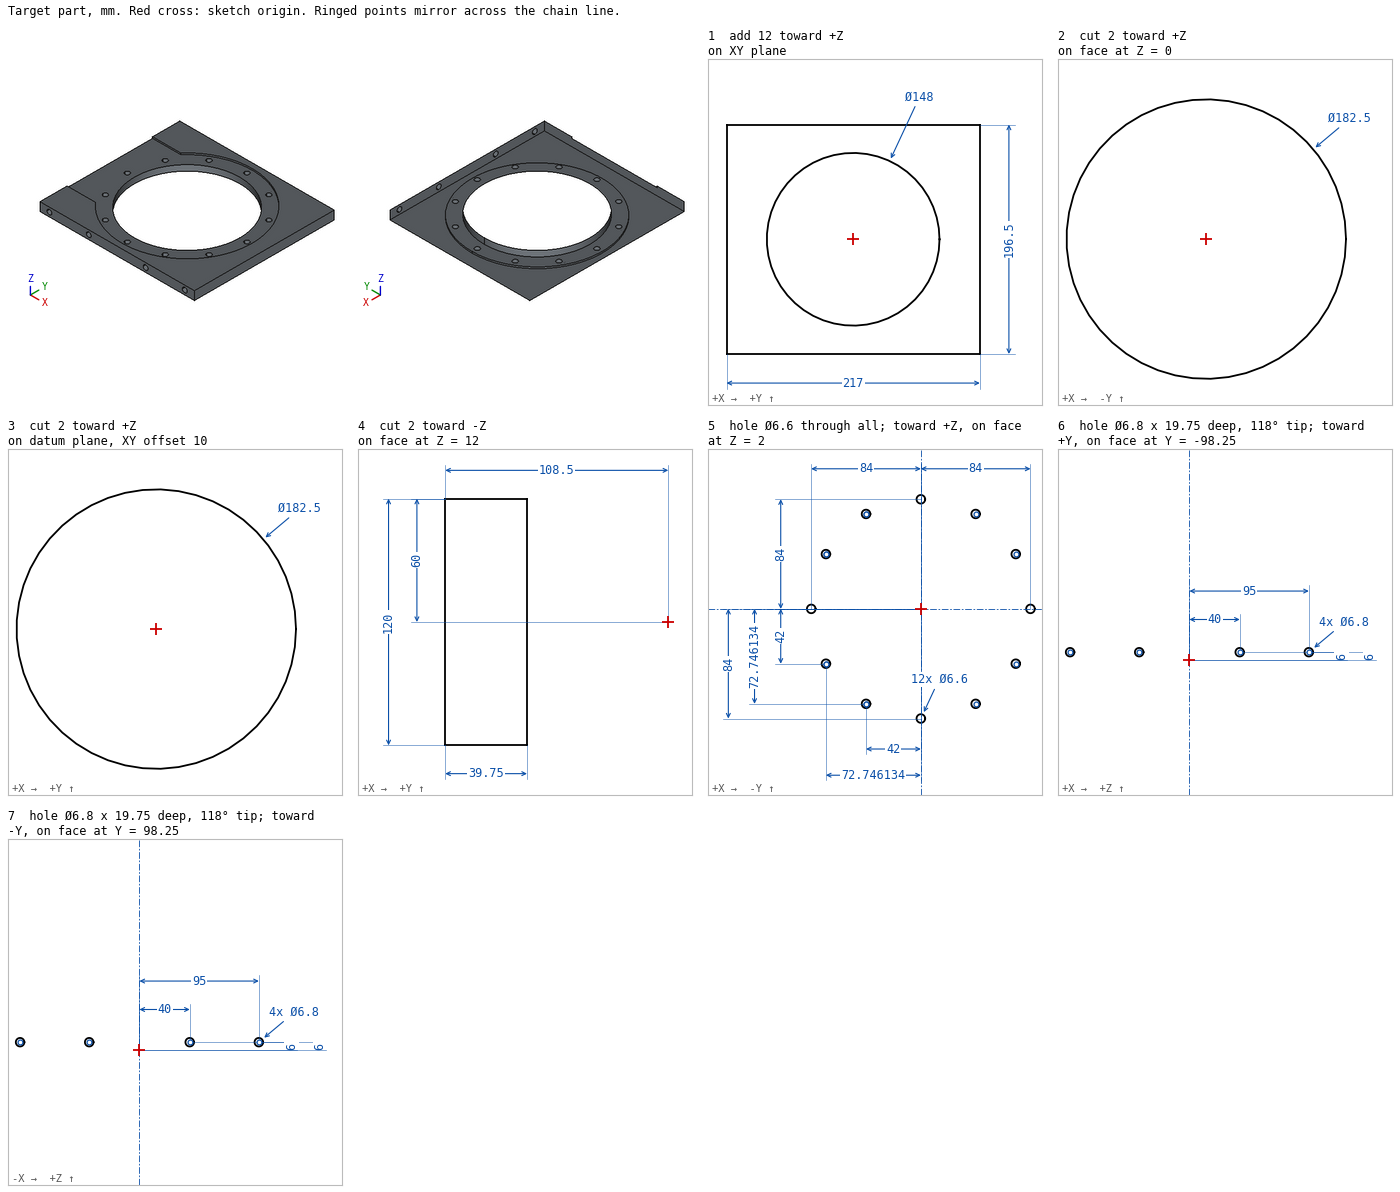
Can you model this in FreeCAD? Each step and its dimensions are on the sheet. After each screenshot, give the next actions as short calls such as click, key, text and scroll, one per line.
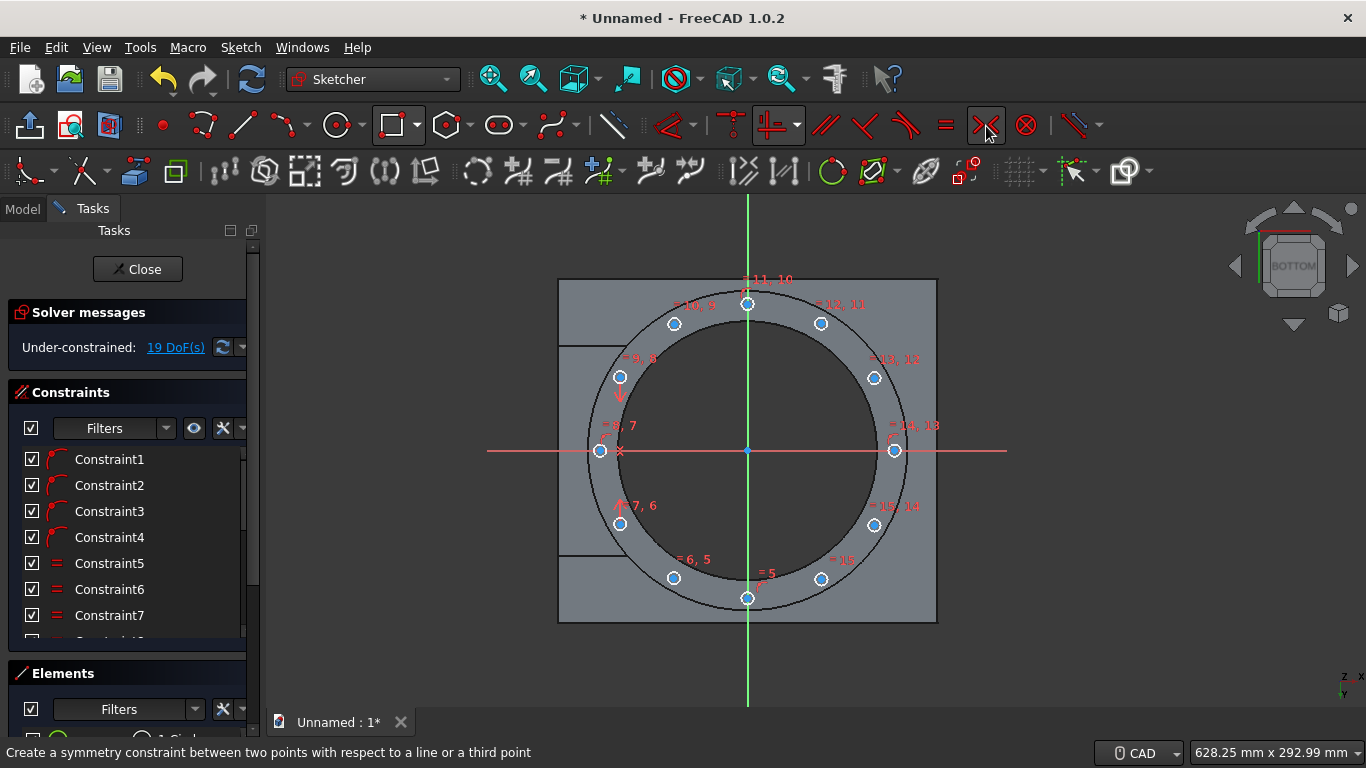
click(674, 578)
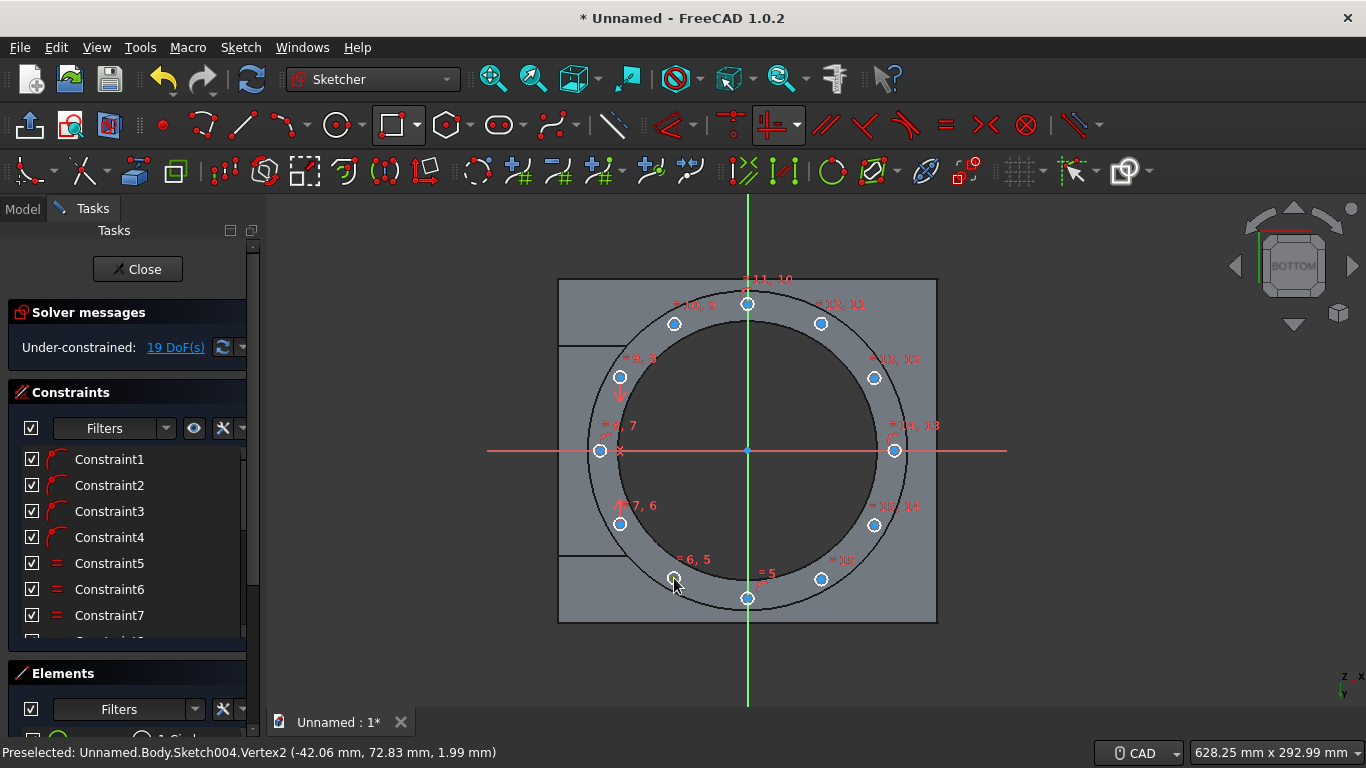
click(674, 324)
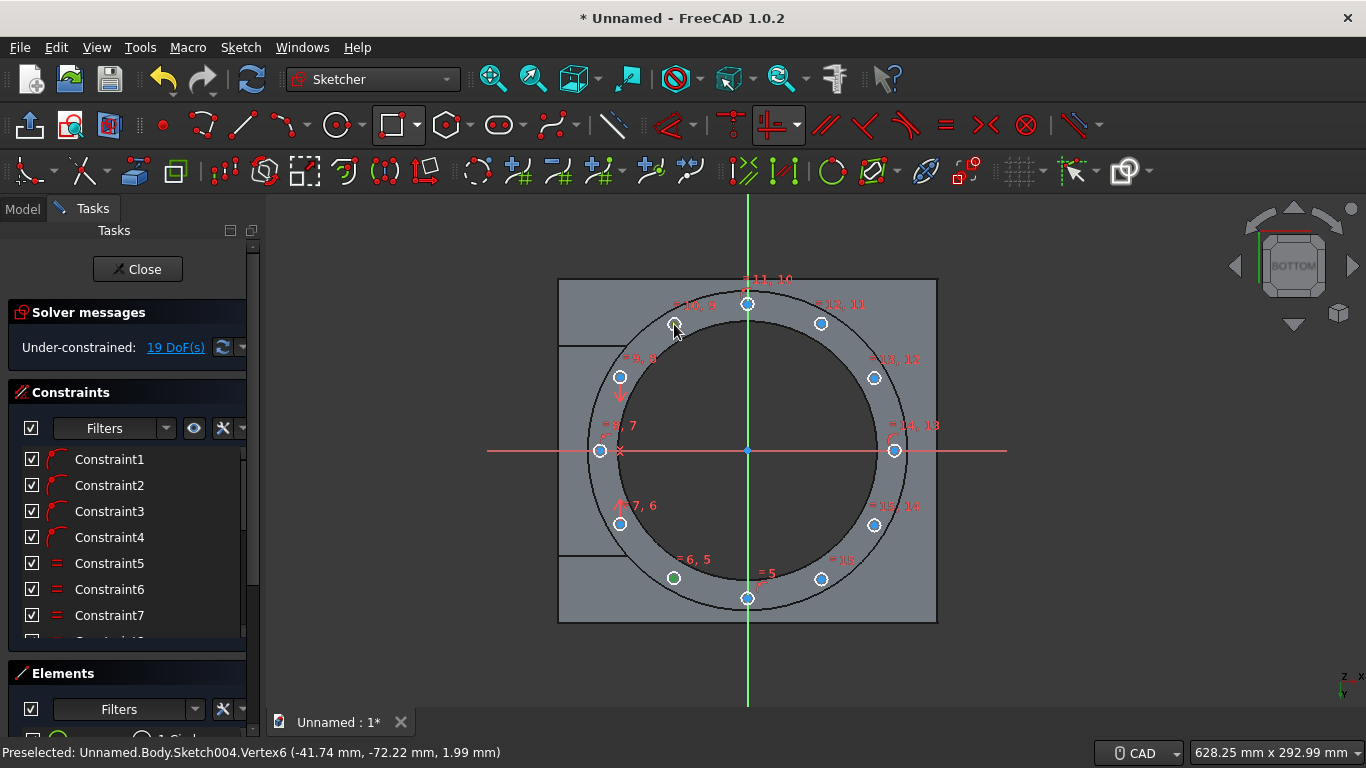
click(488, 451)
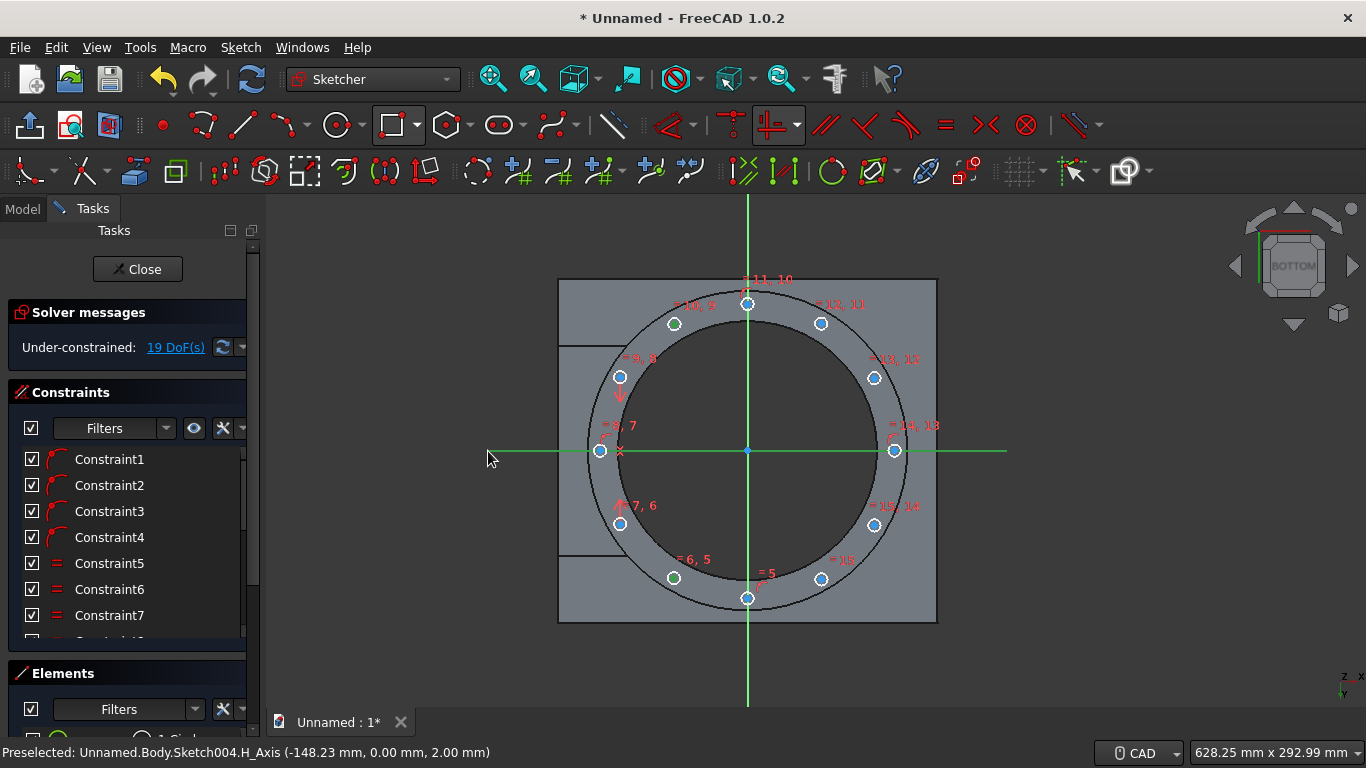
click(986, 126)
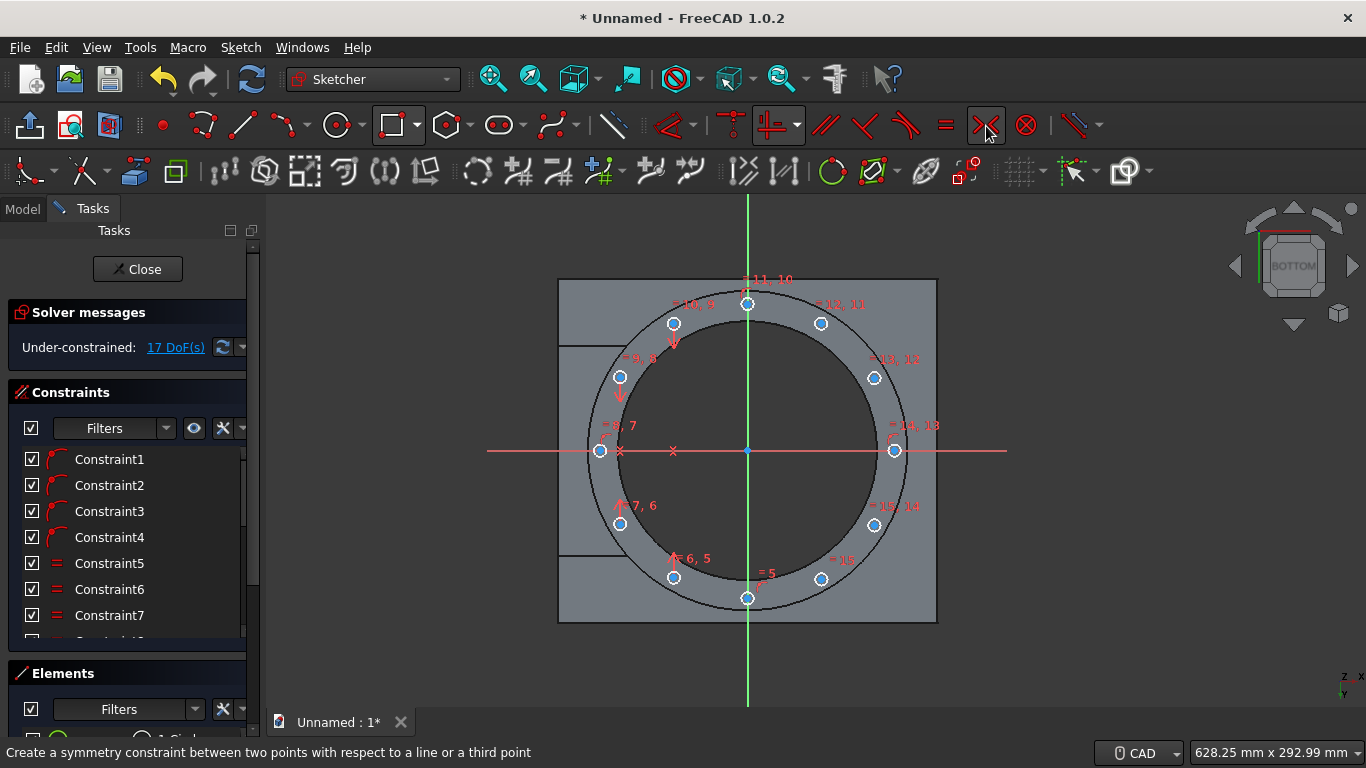
click(674, 324)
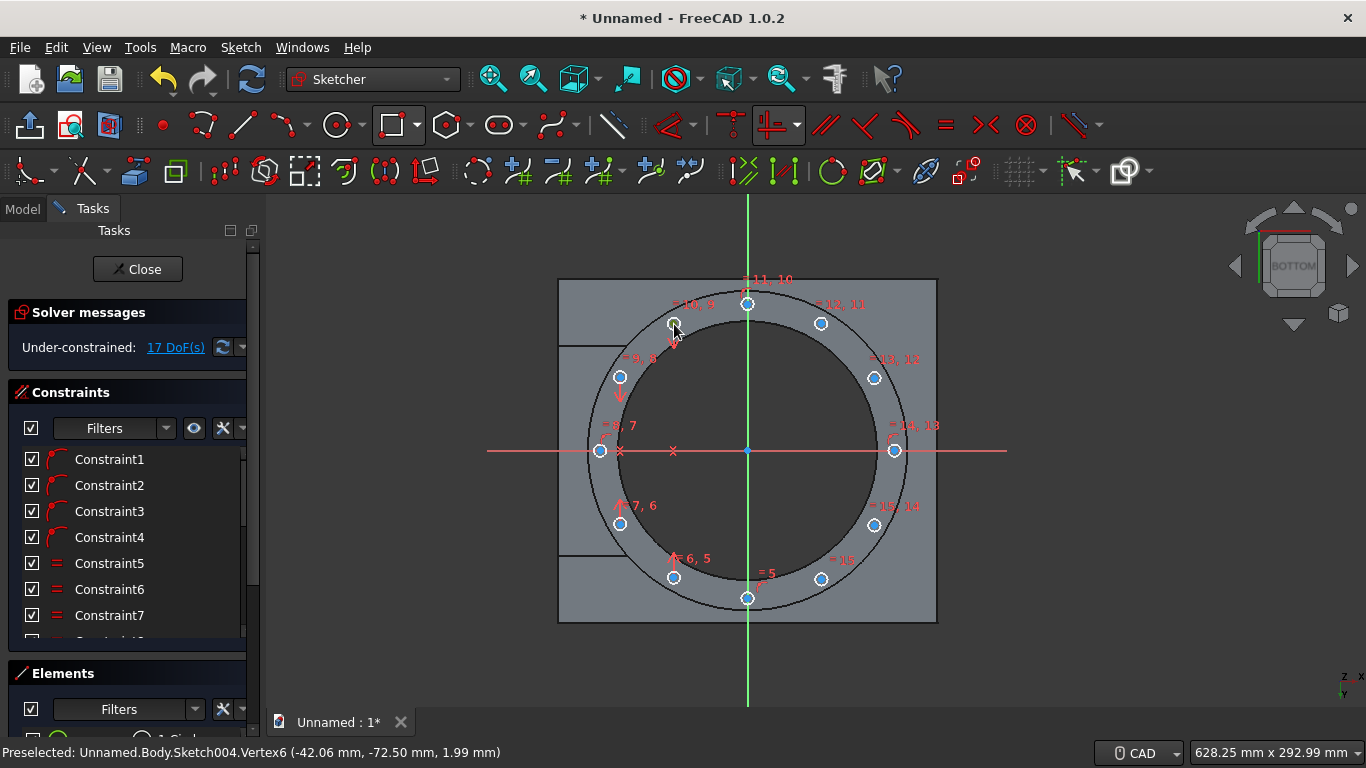
click(821, 324)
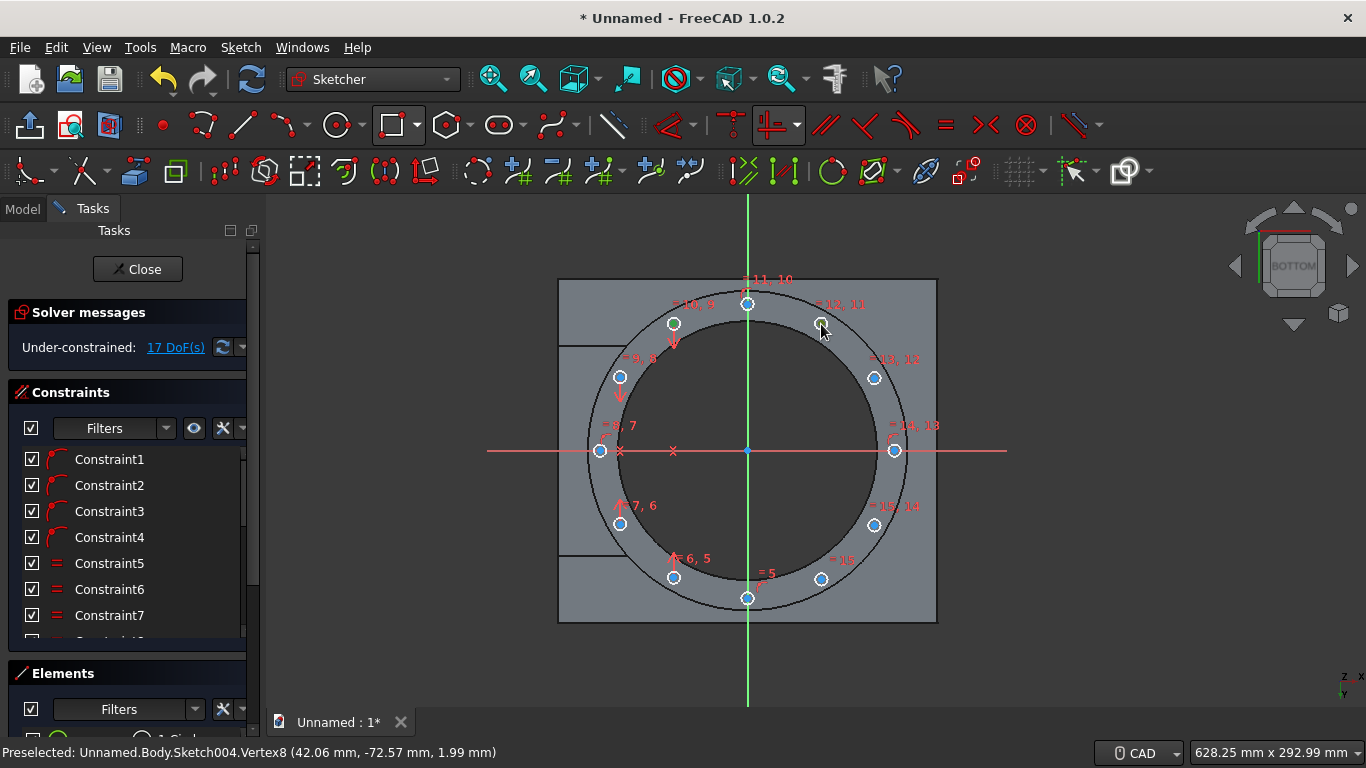
click(748, 646)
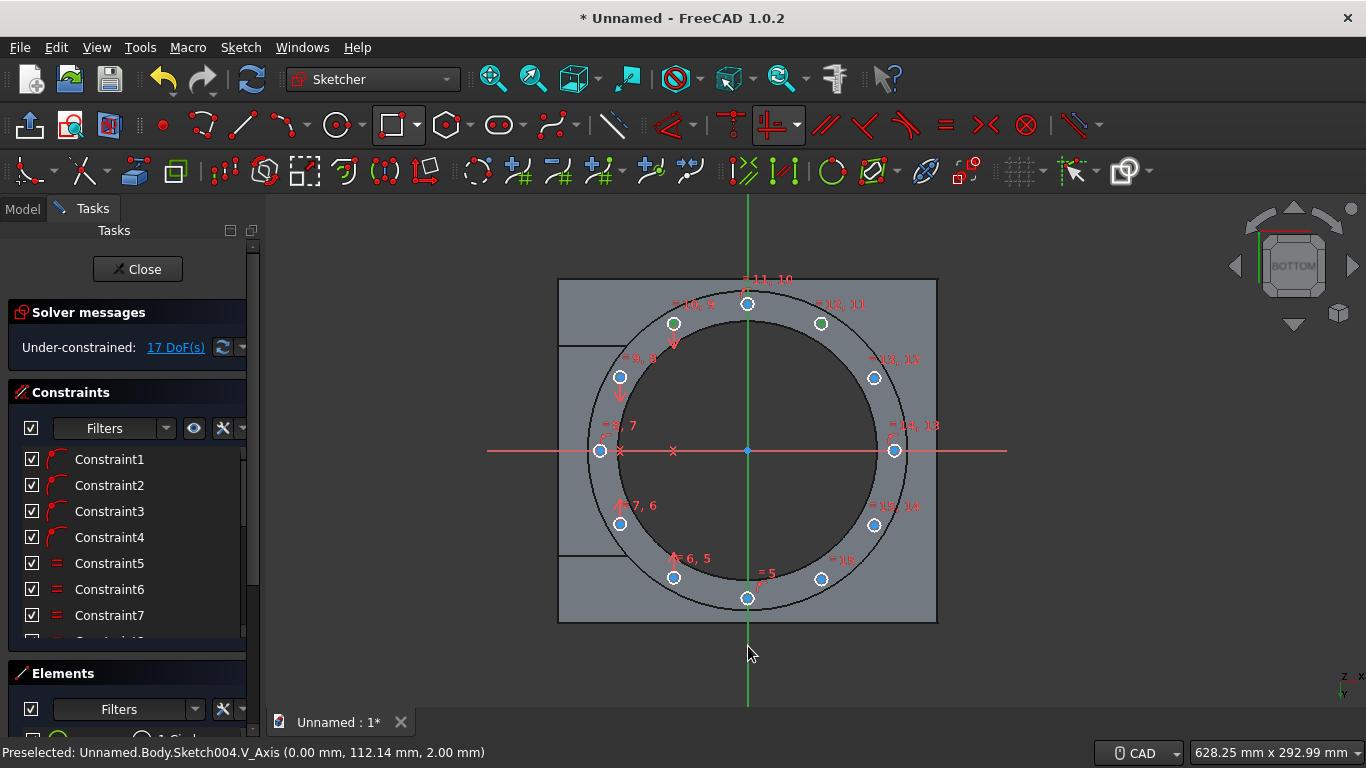
click(986, 126)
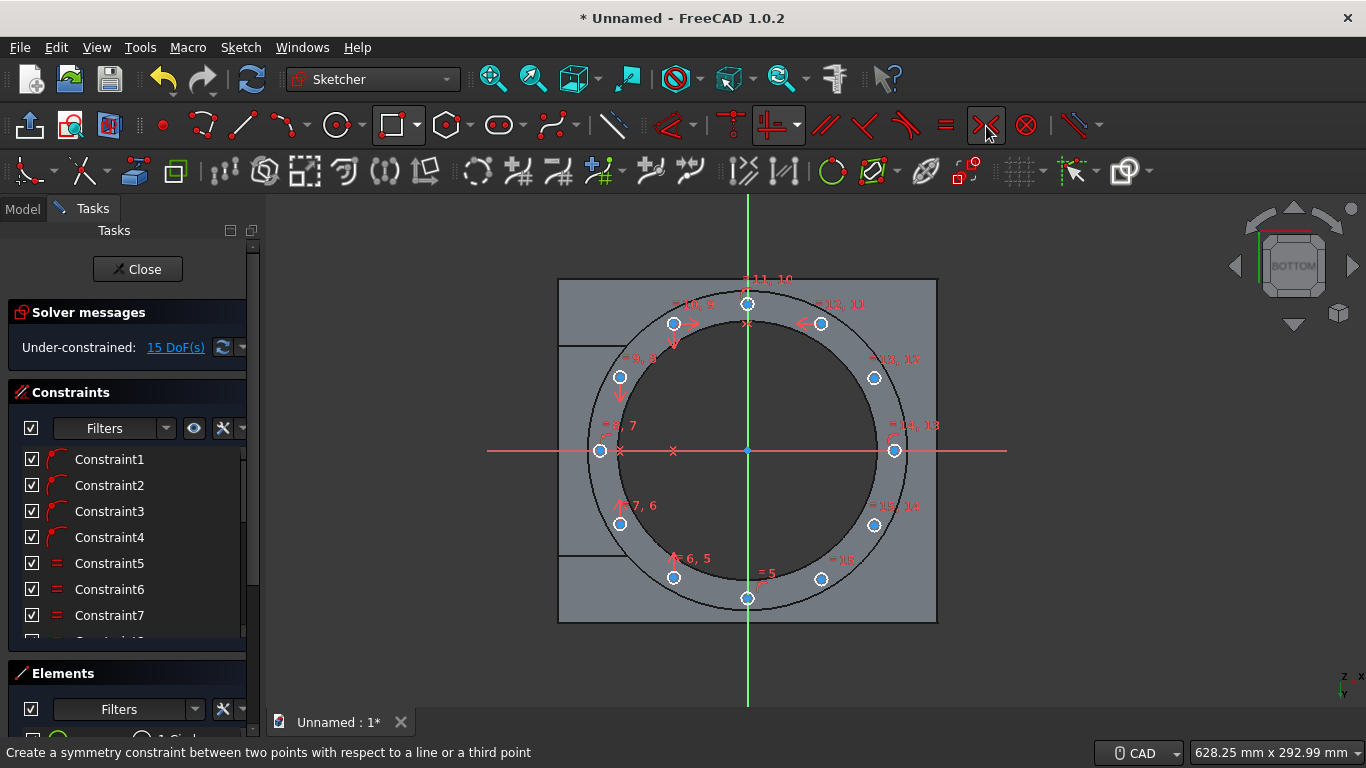
click(620, 377)